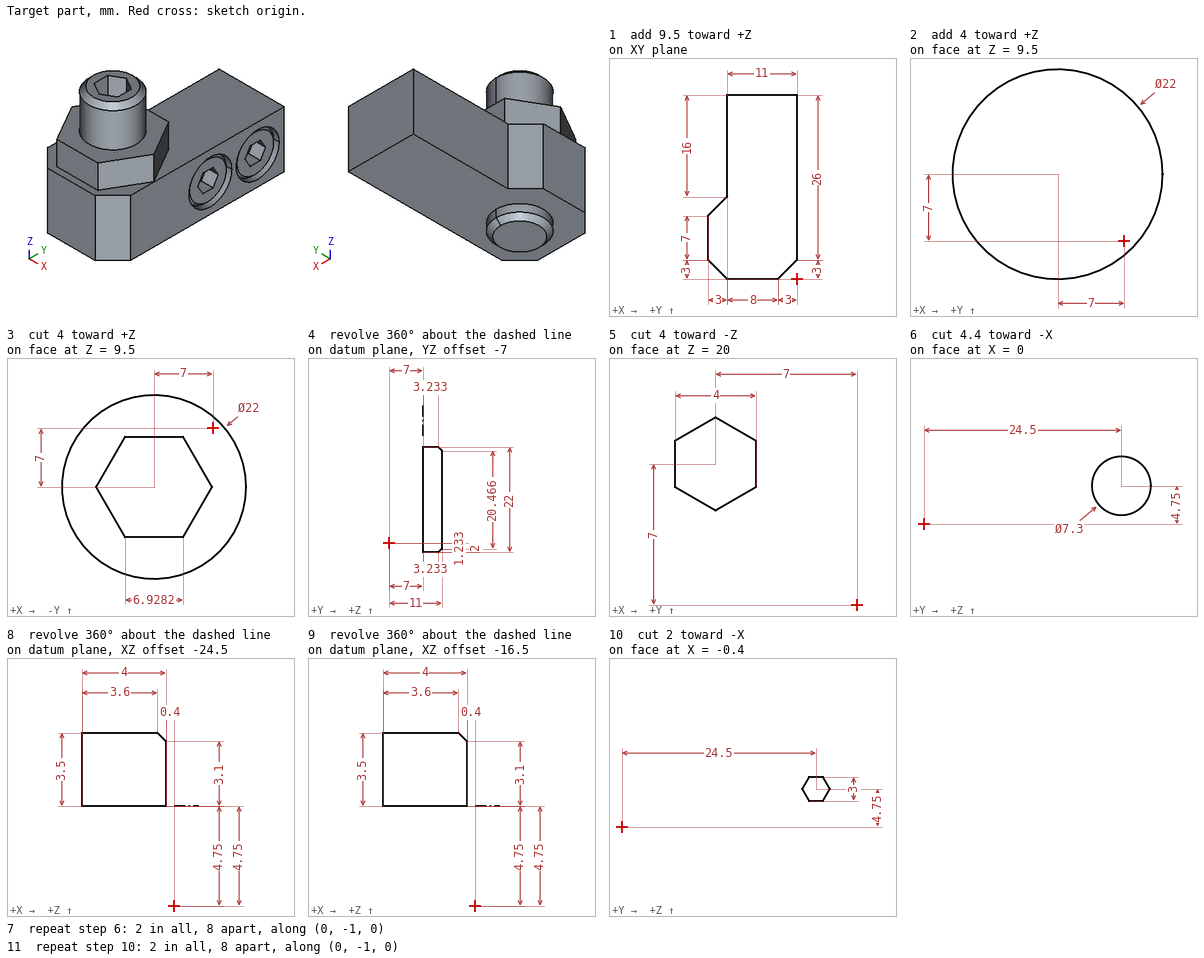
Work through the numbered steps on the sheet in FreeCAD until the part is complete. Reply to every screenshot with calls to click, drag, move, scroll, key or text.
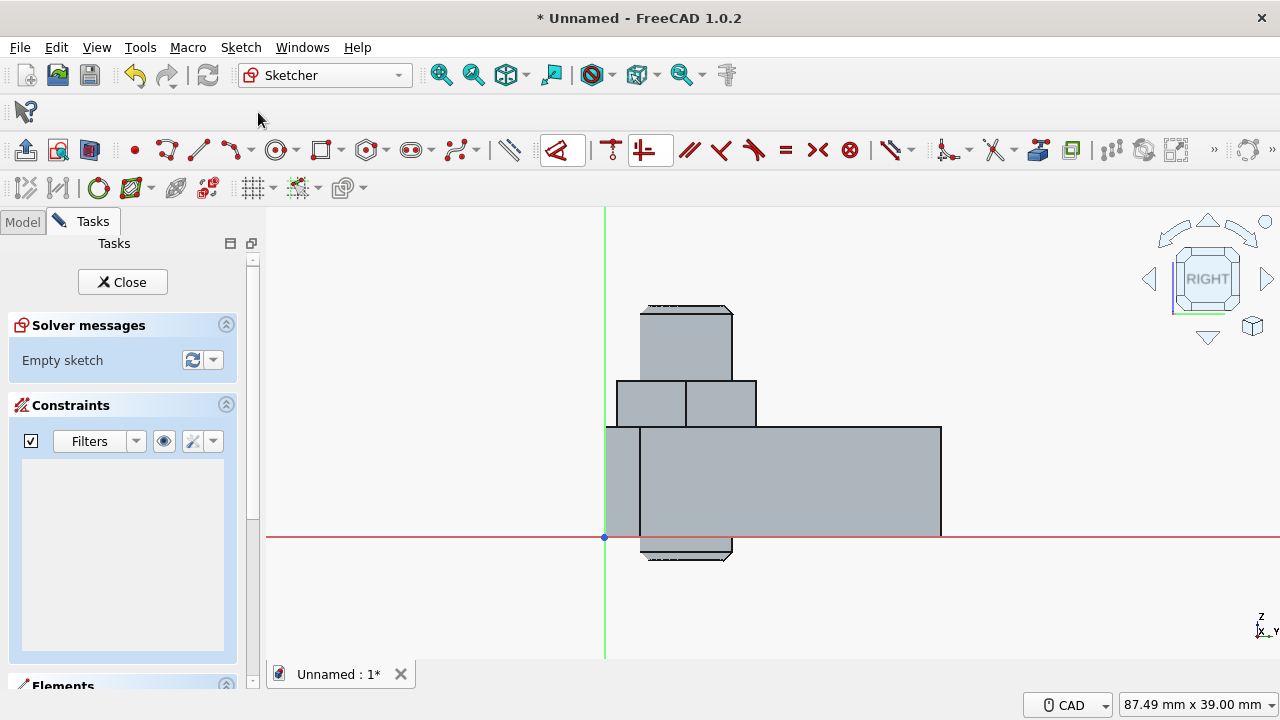
scroll(968, 503, up, 6)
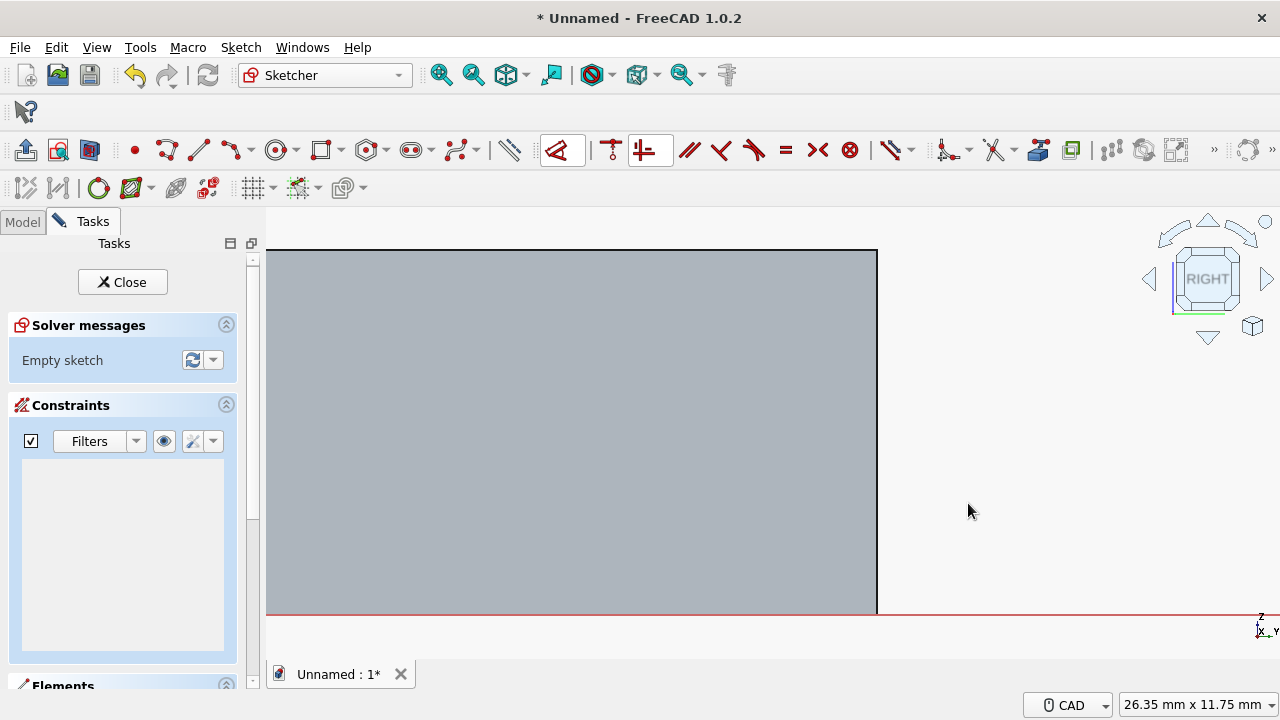
key(g)
key(c)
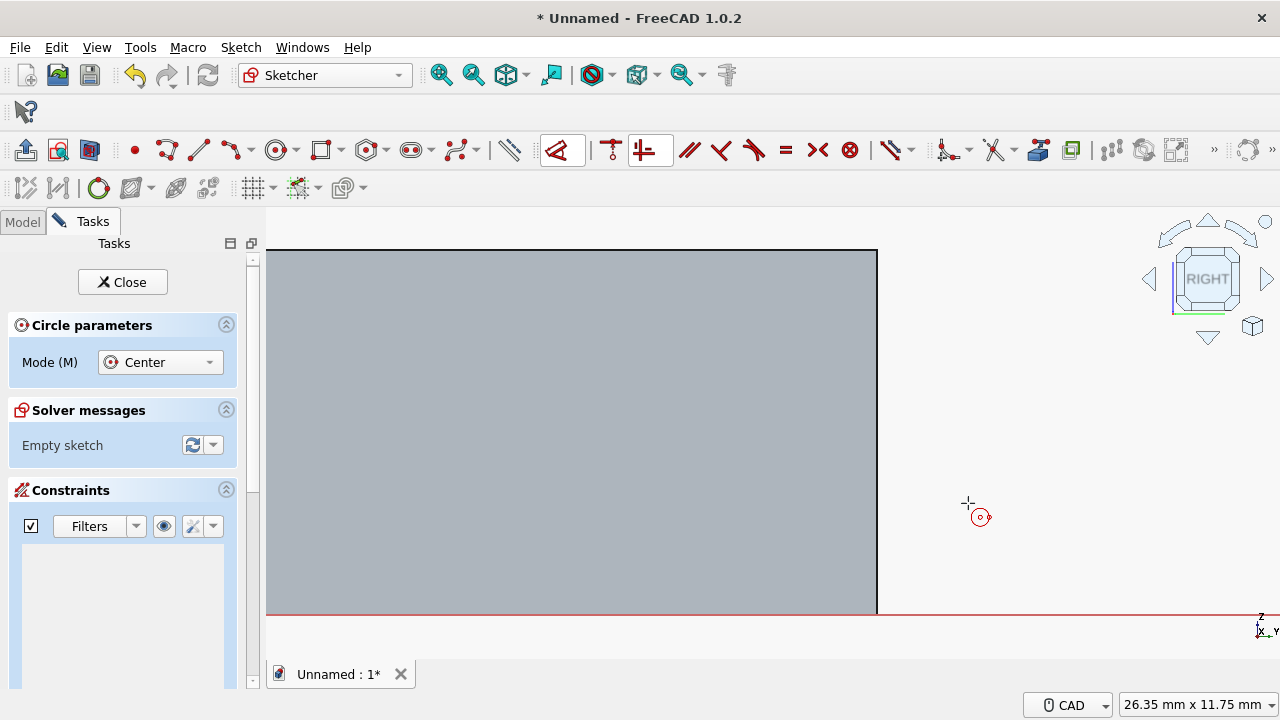
click(704, 433)
click(803, 333)
key(Escape)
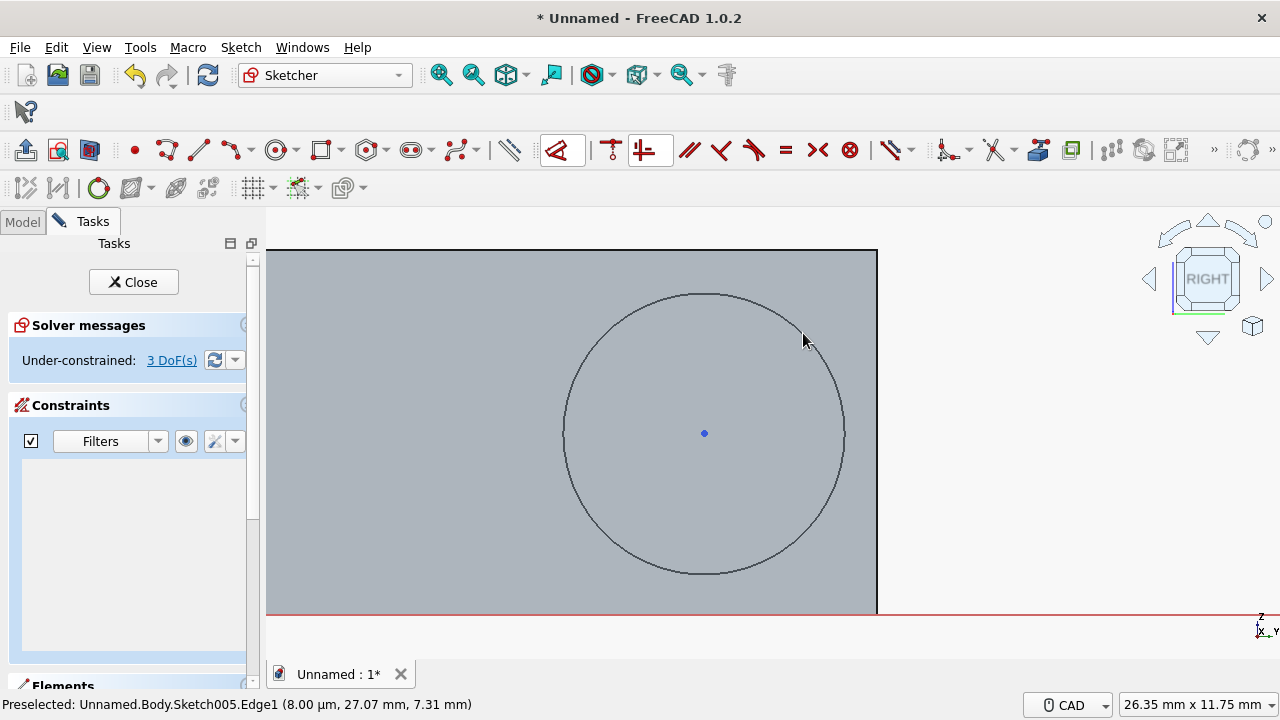
click(803, 334)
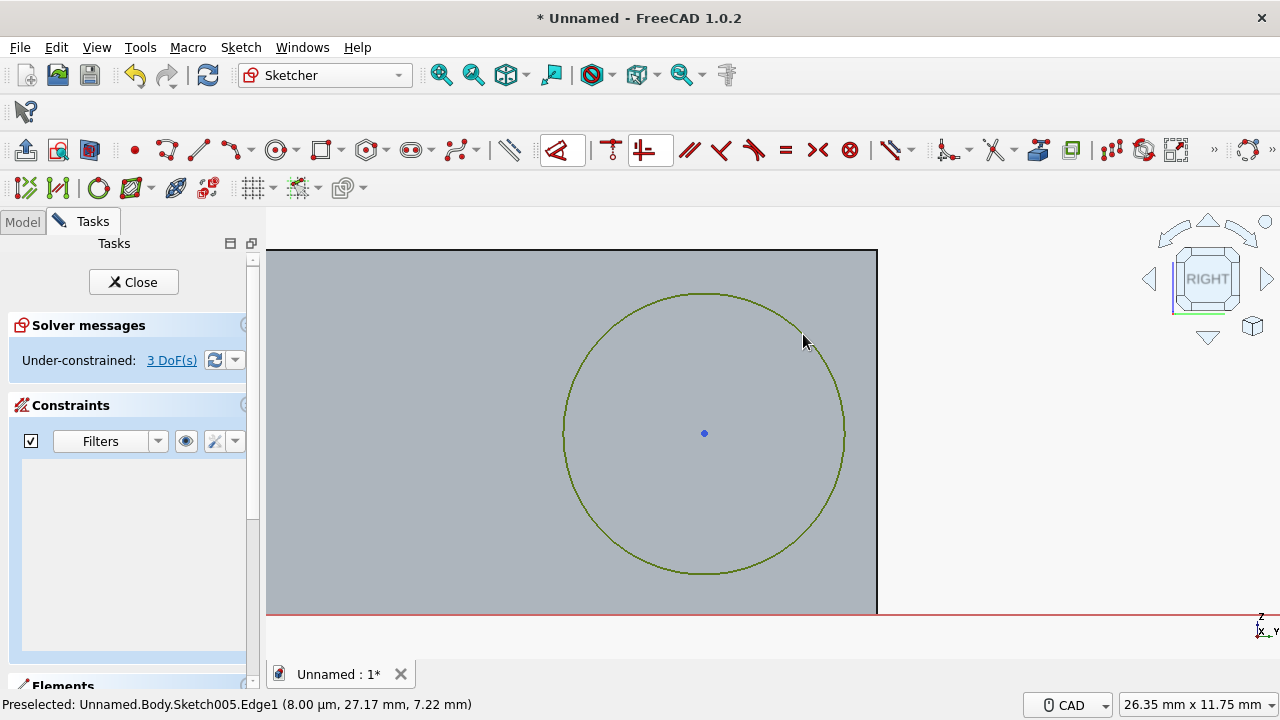
click(580, 150)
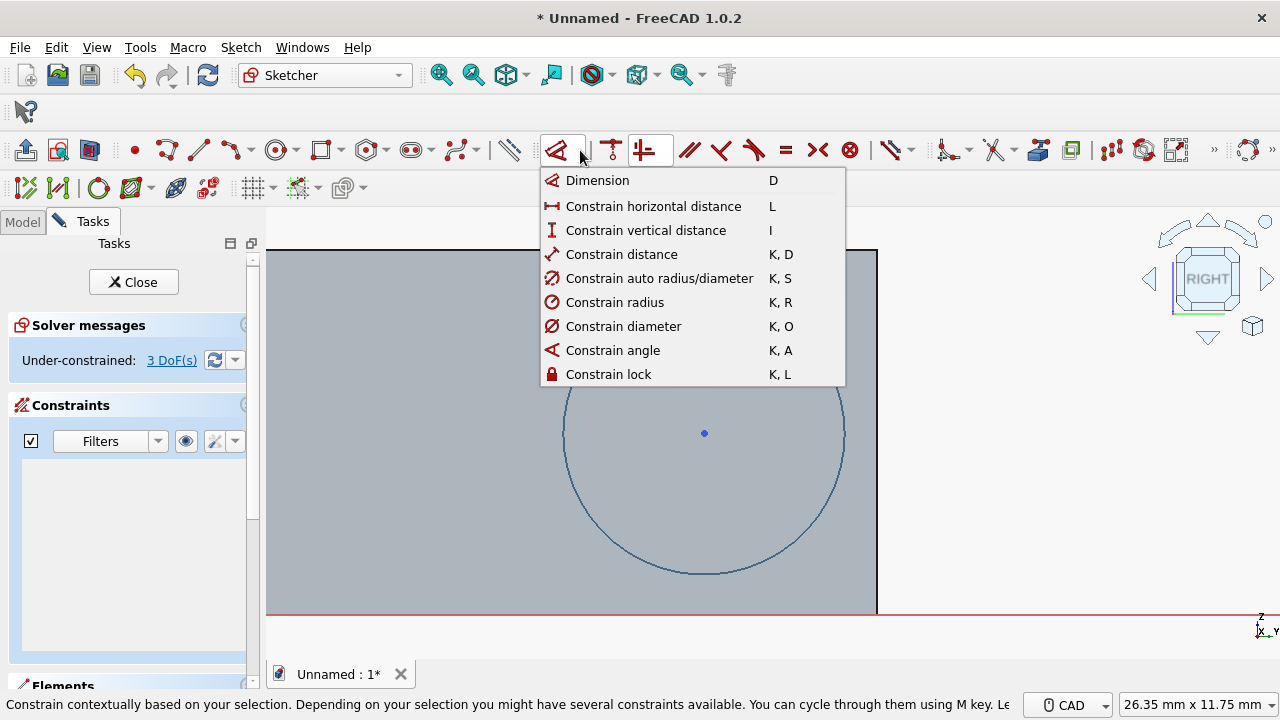
click(693, 326)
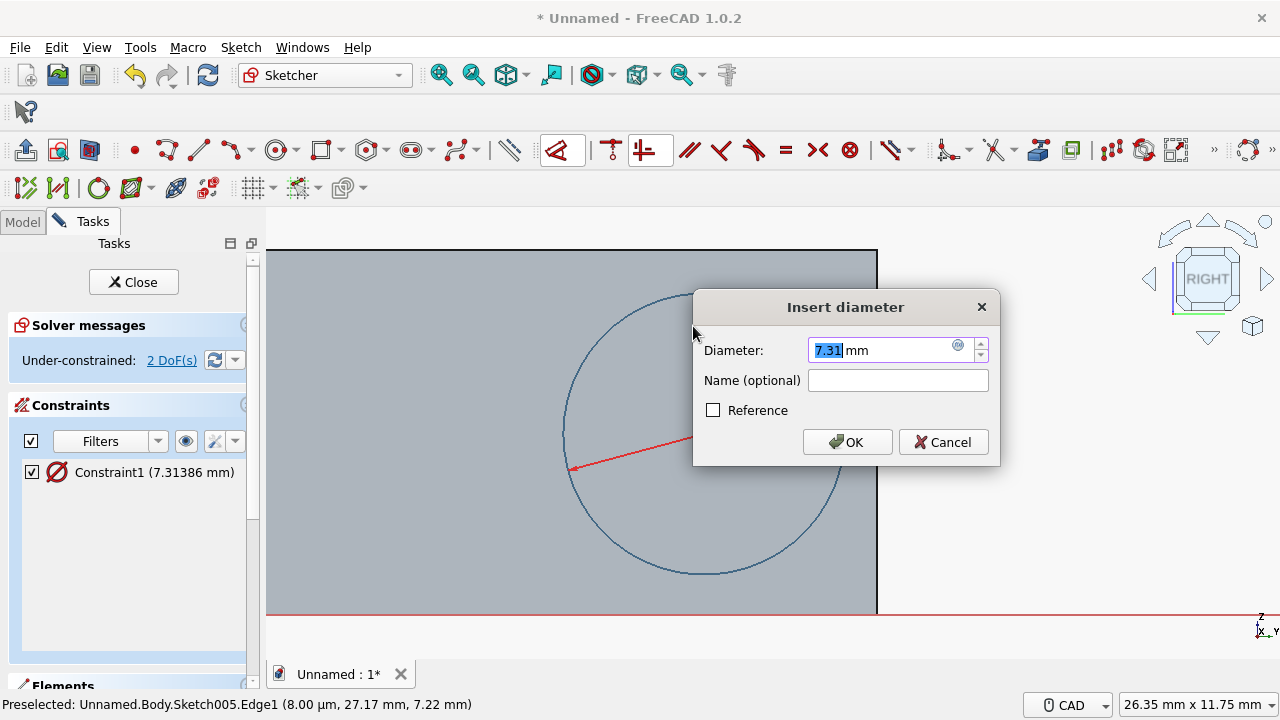
text(7.3)
key(Return)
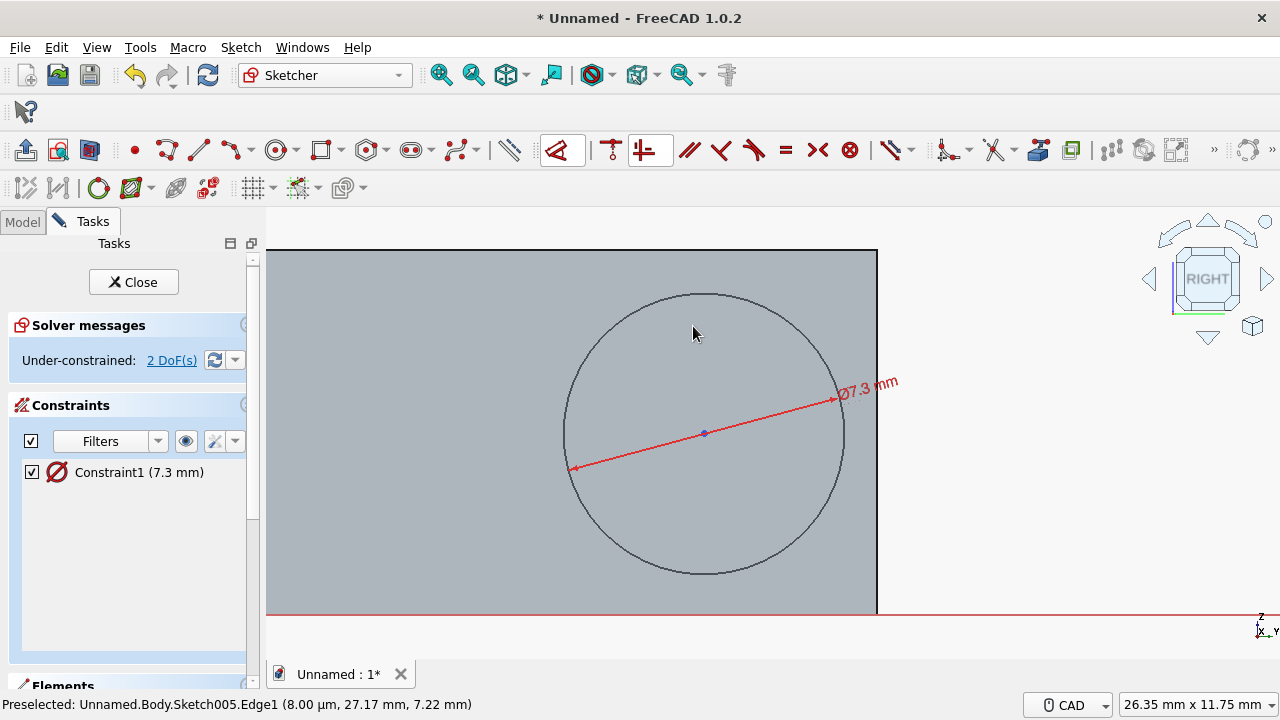
click(704, 434)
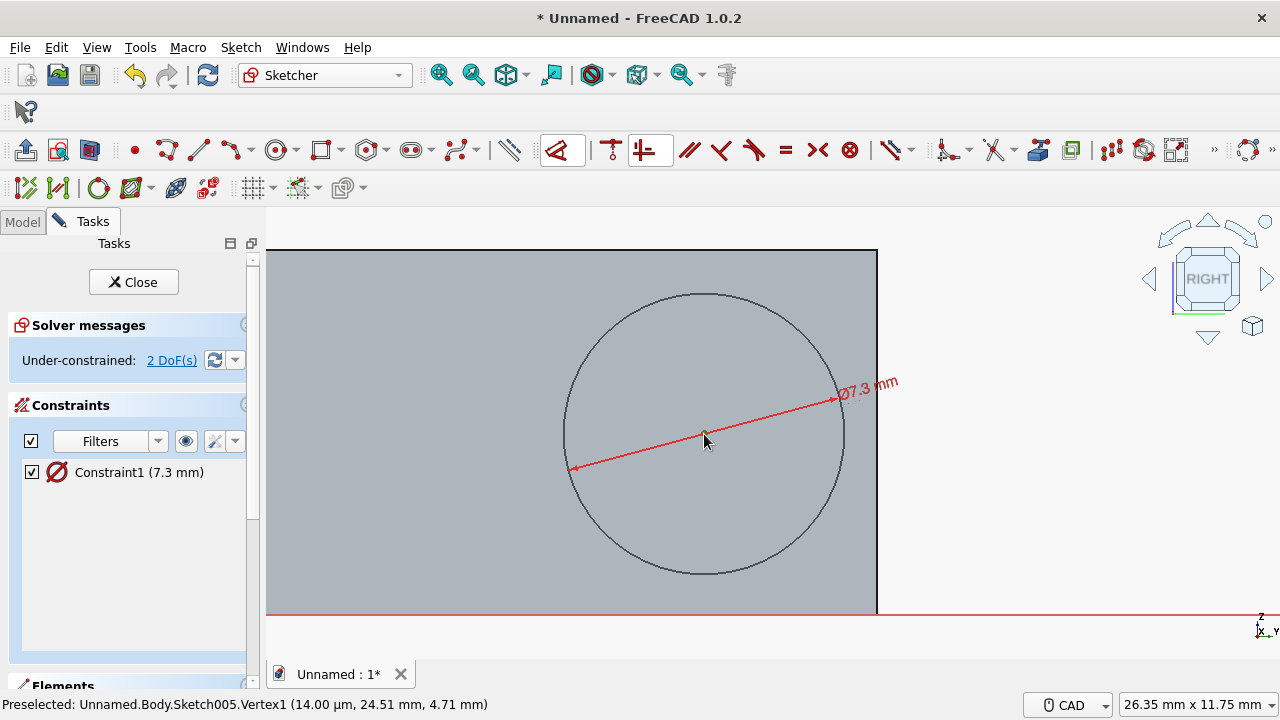
click(580, 150)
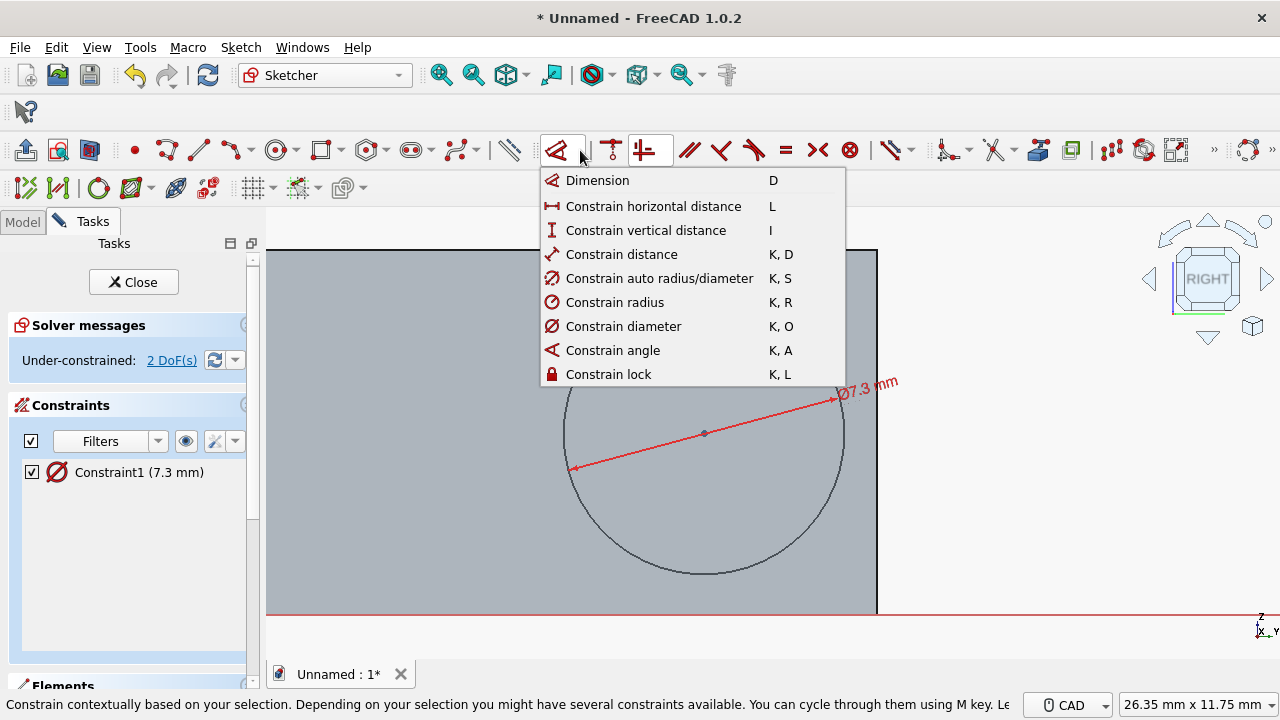
click(693, 206)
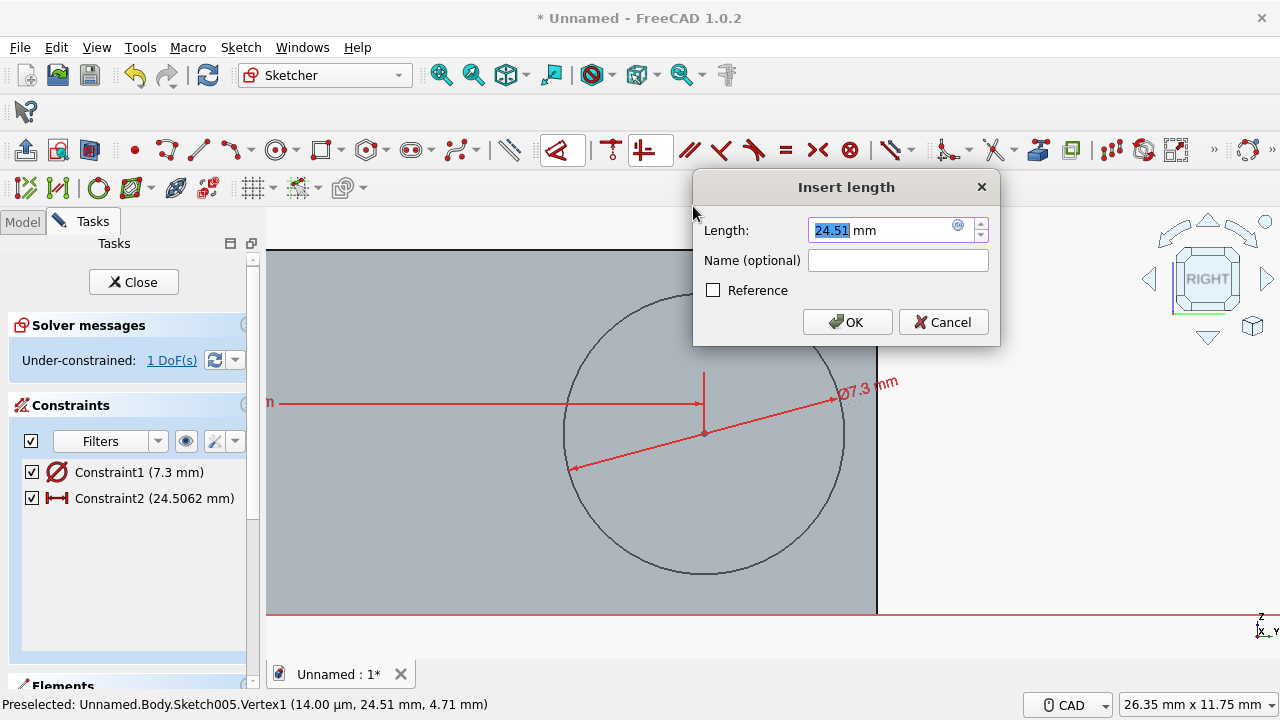
text(24.5)
key(Return)